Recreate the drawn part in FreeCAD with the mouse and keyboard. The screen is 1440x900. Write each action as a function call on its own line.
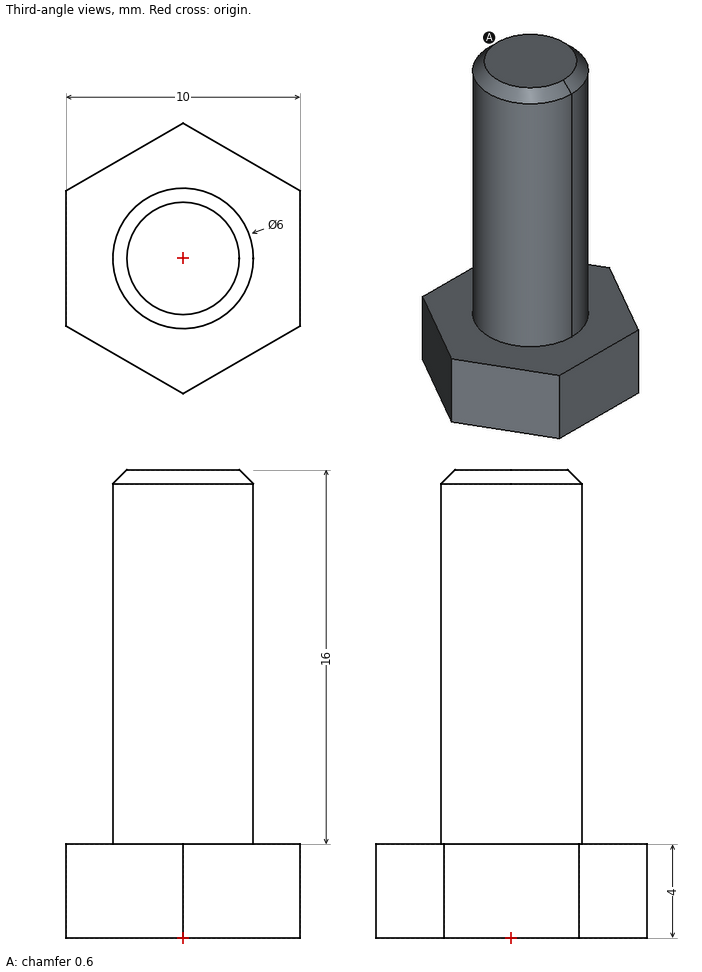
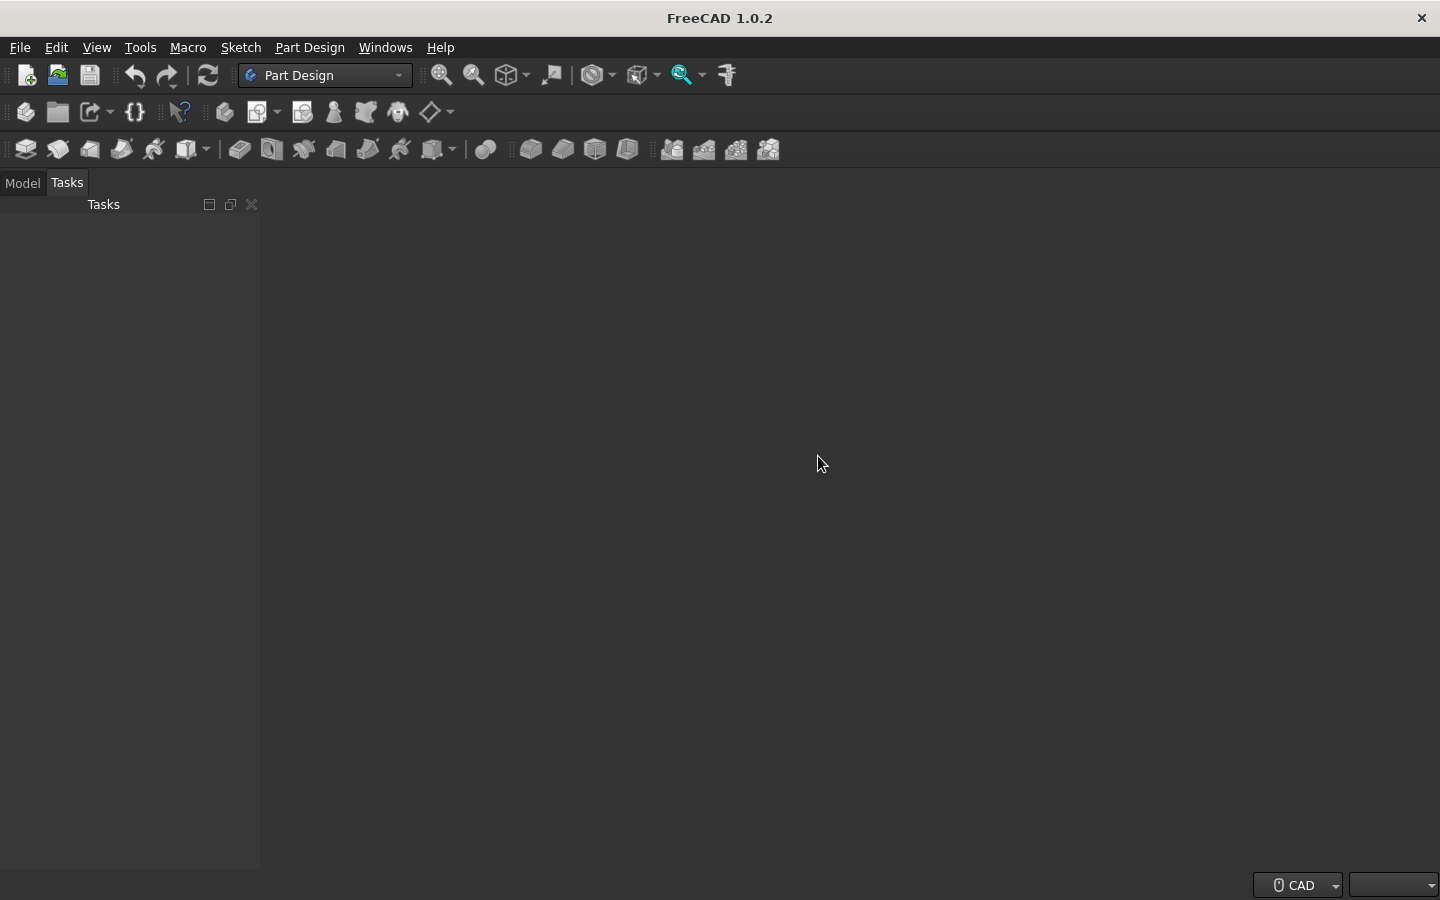
key(ctrl+n)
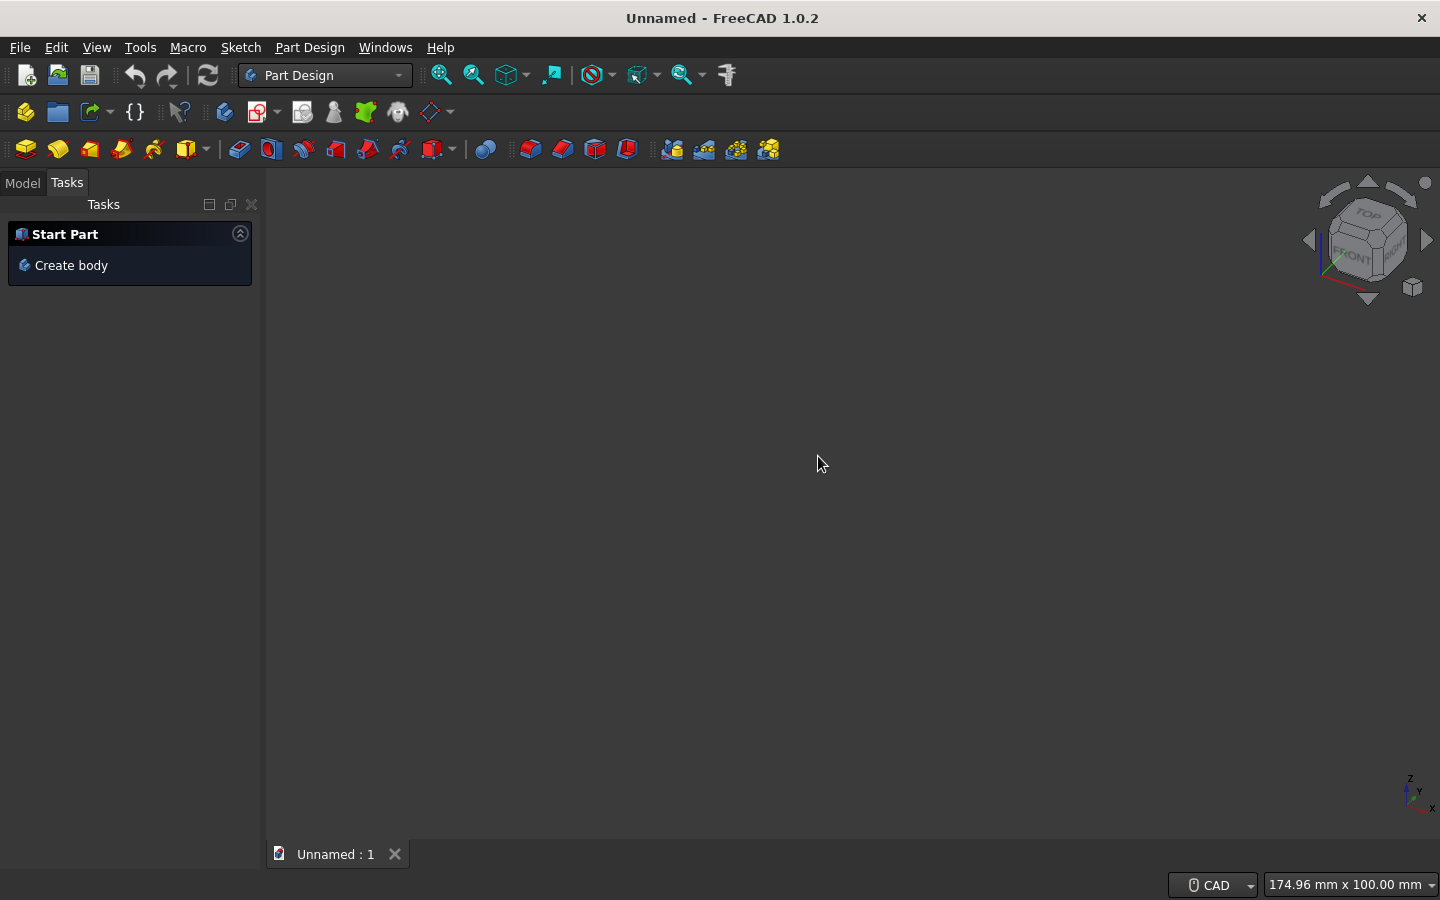
click(258, 112)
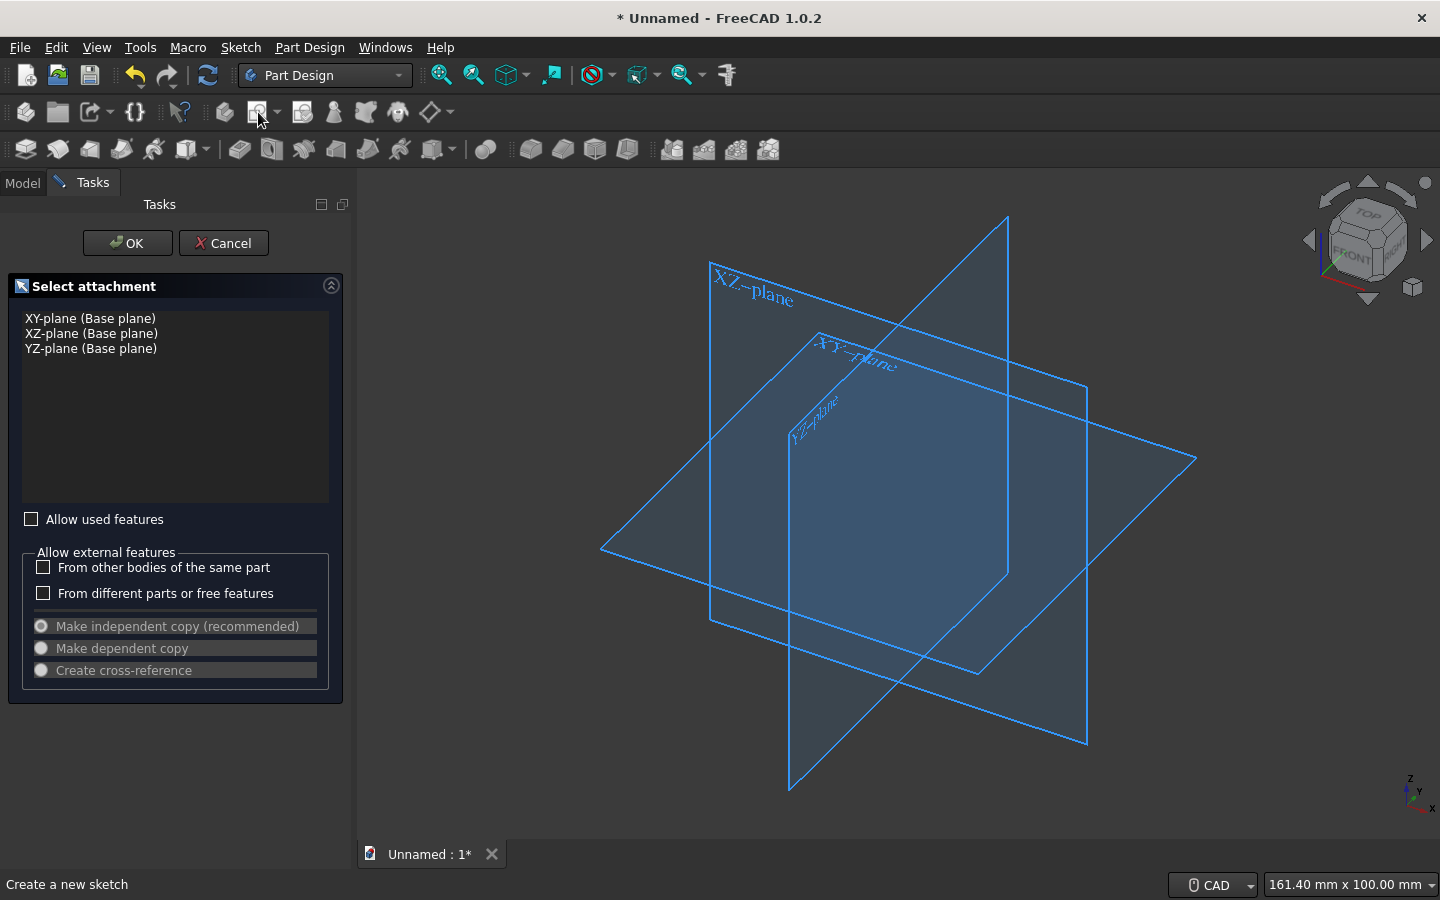
click(82, 318)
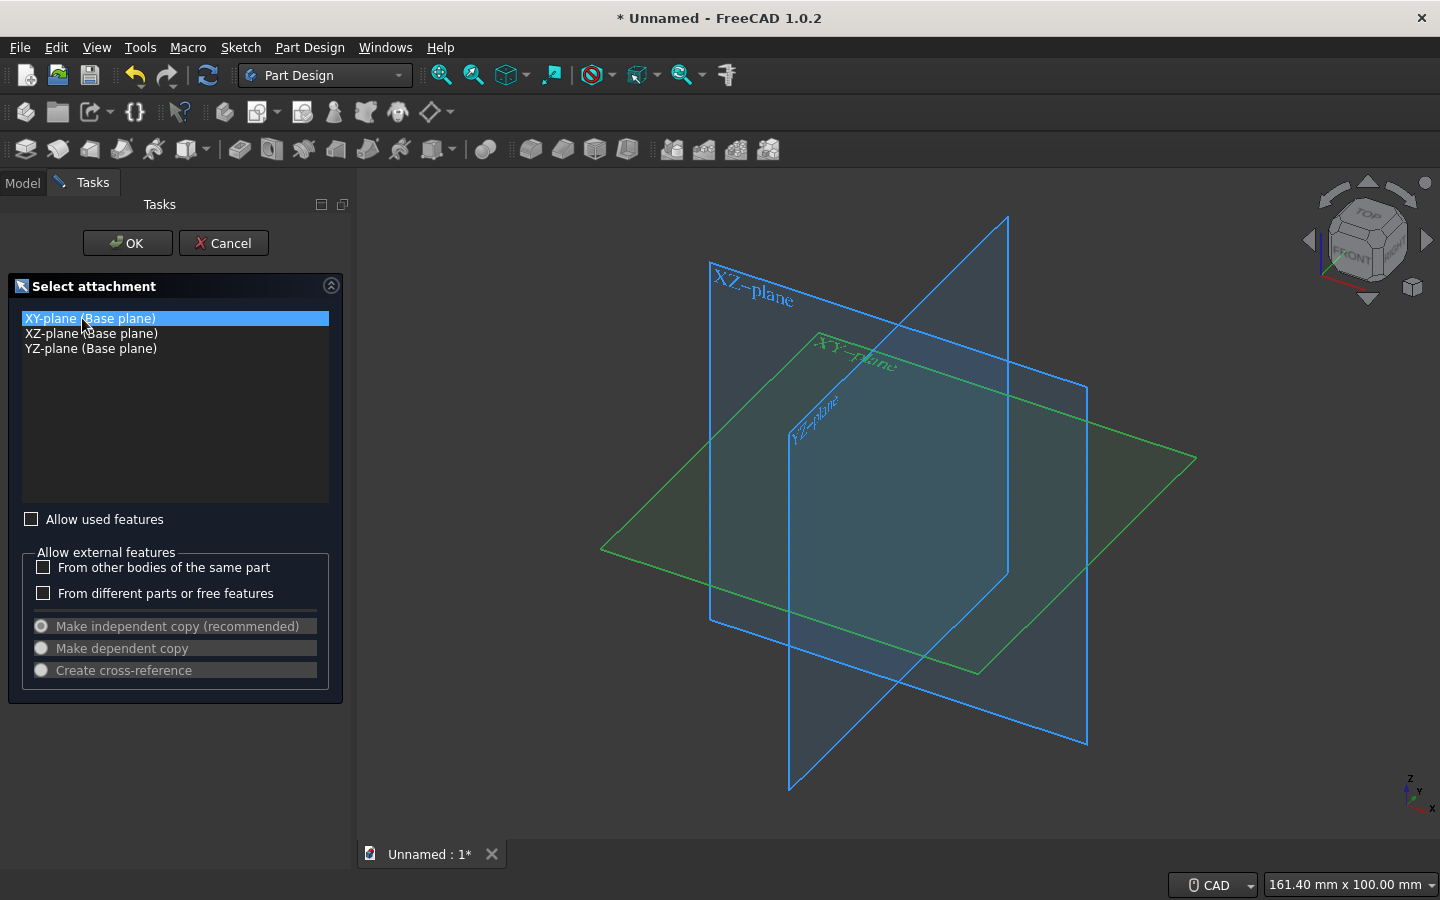
click(128, 243)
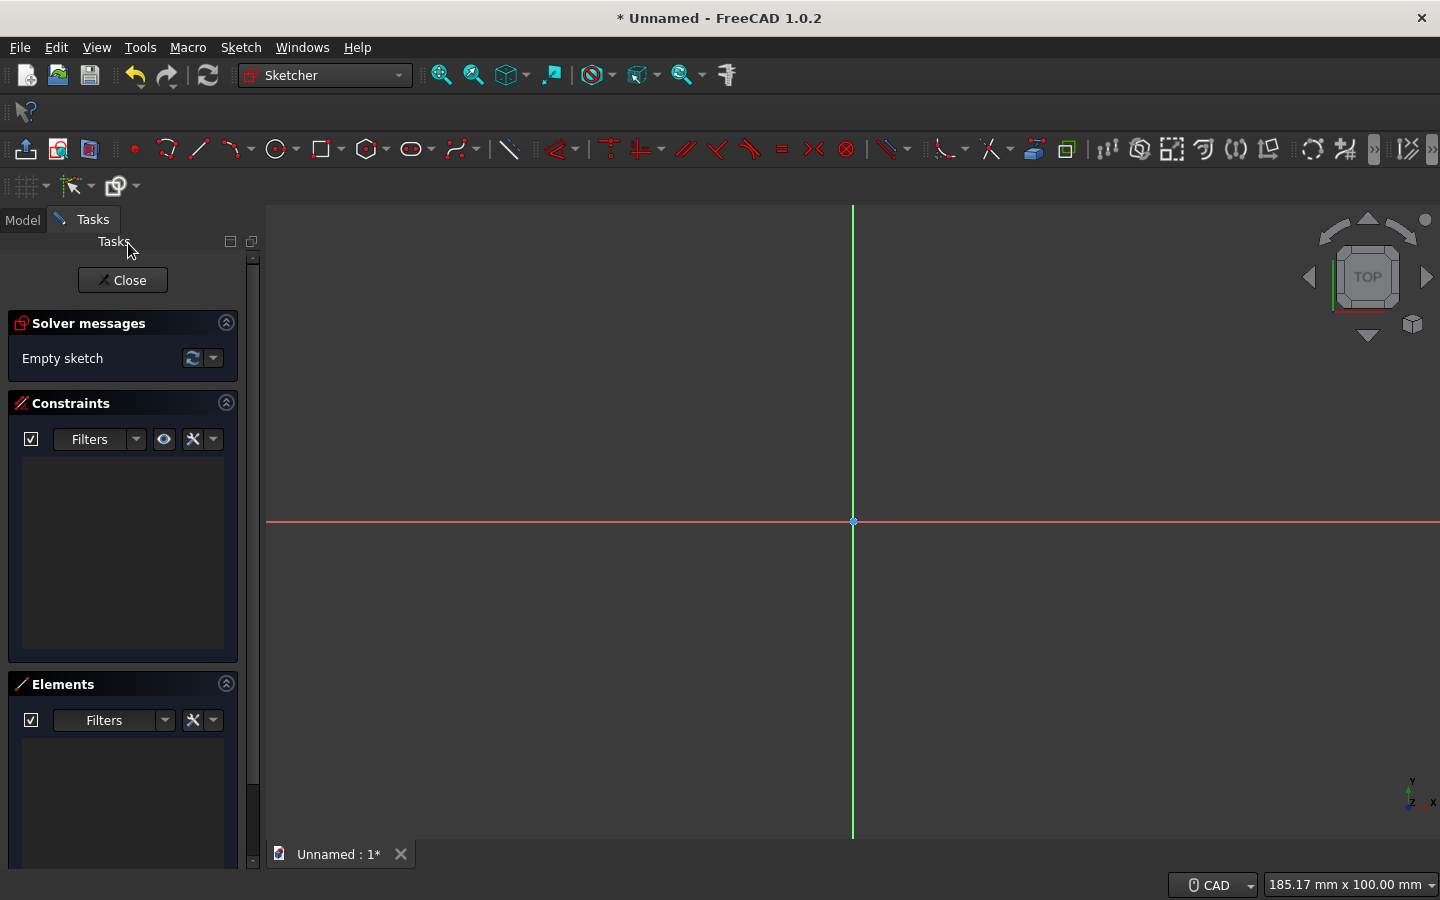
scroll(867, 522, up, 9)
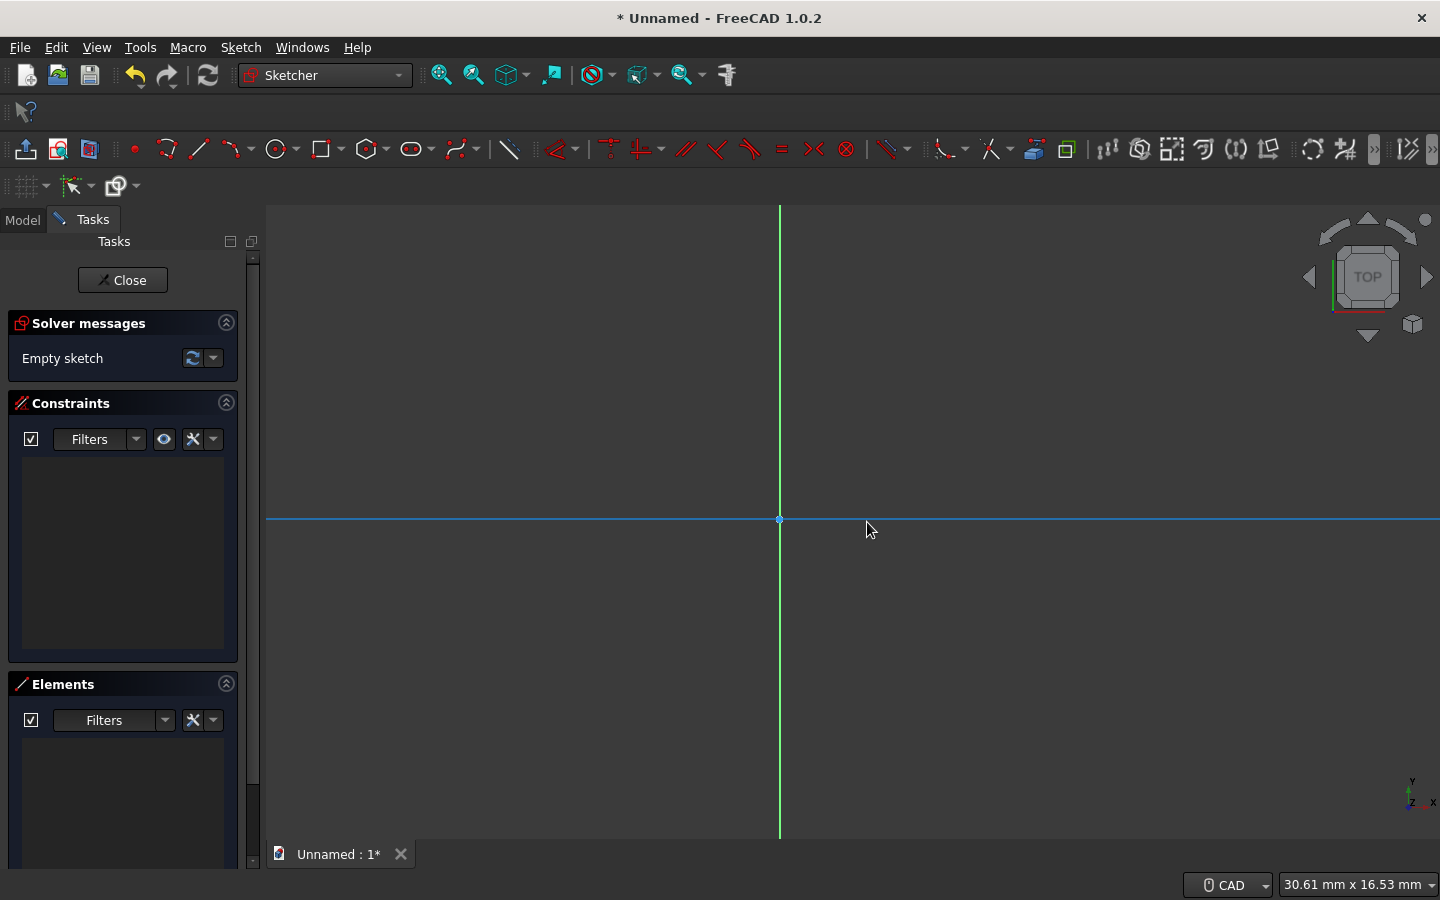
click(366, 150)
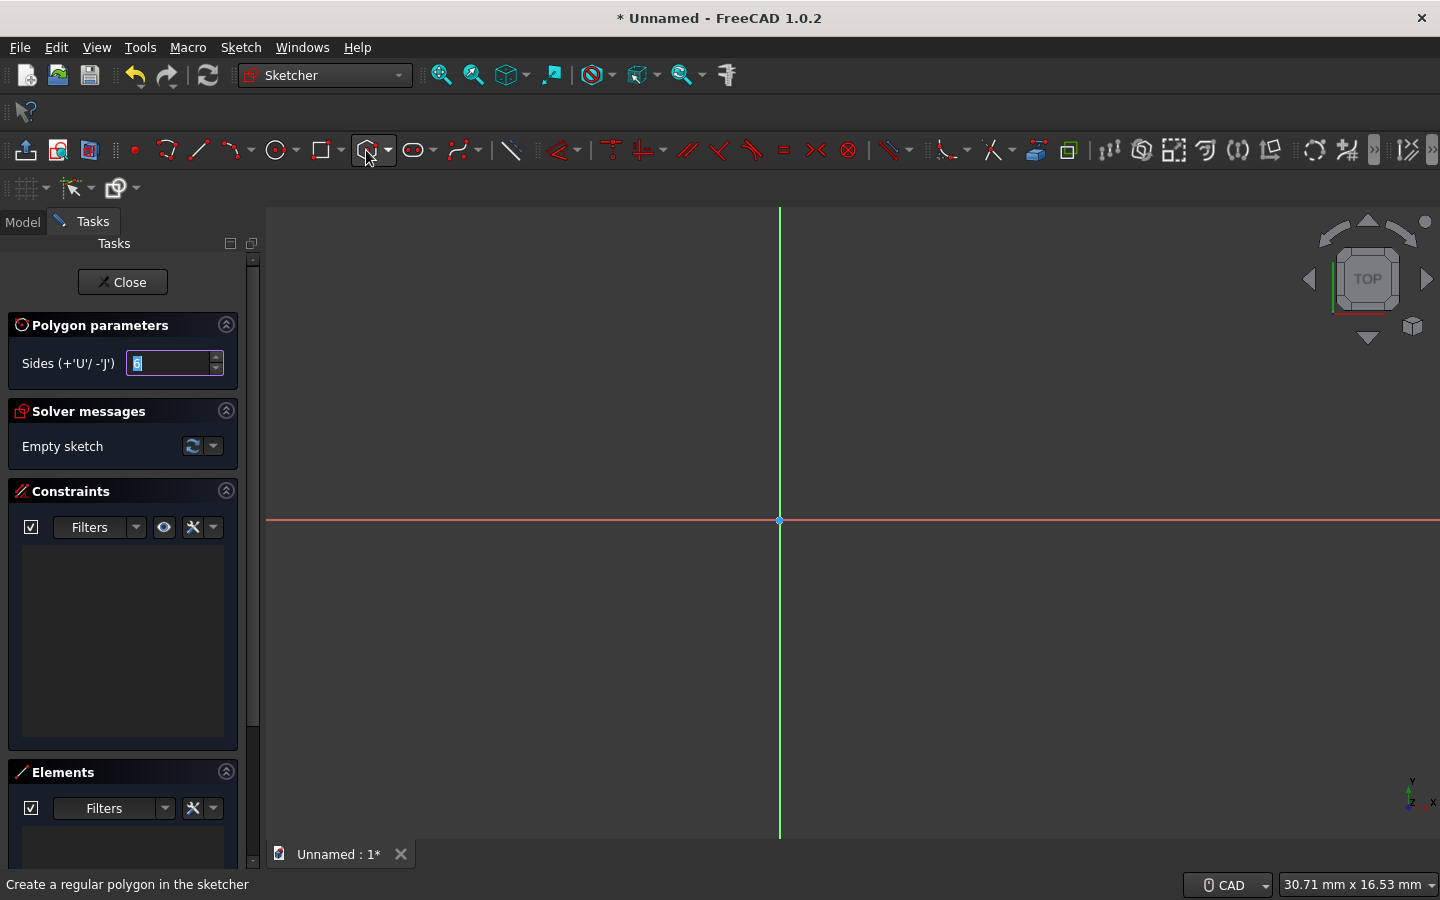
click(780, 520)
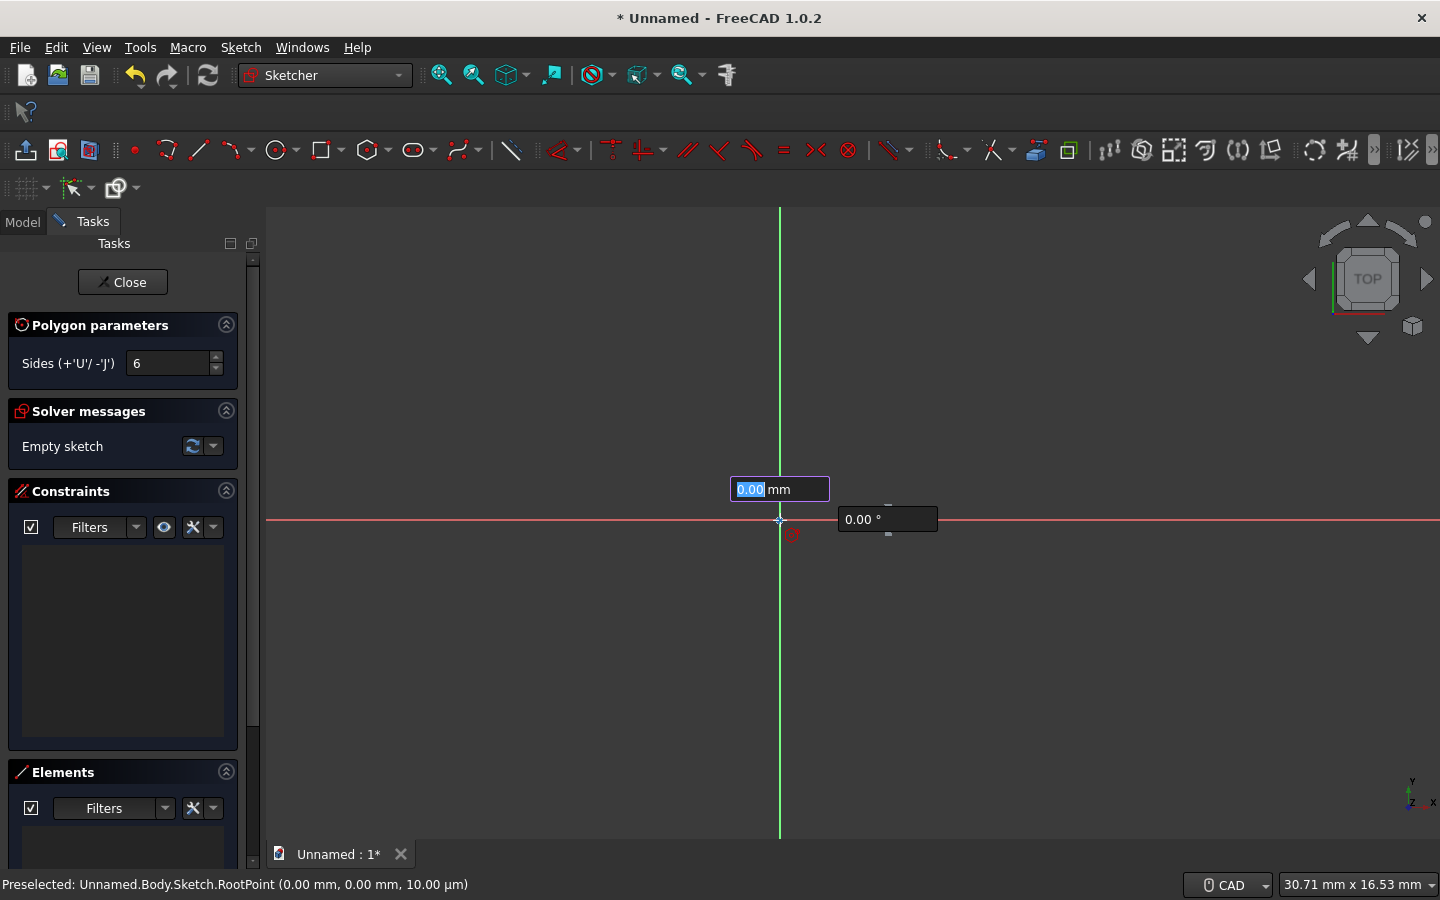
click(780, 300)
right_click(780, 300)